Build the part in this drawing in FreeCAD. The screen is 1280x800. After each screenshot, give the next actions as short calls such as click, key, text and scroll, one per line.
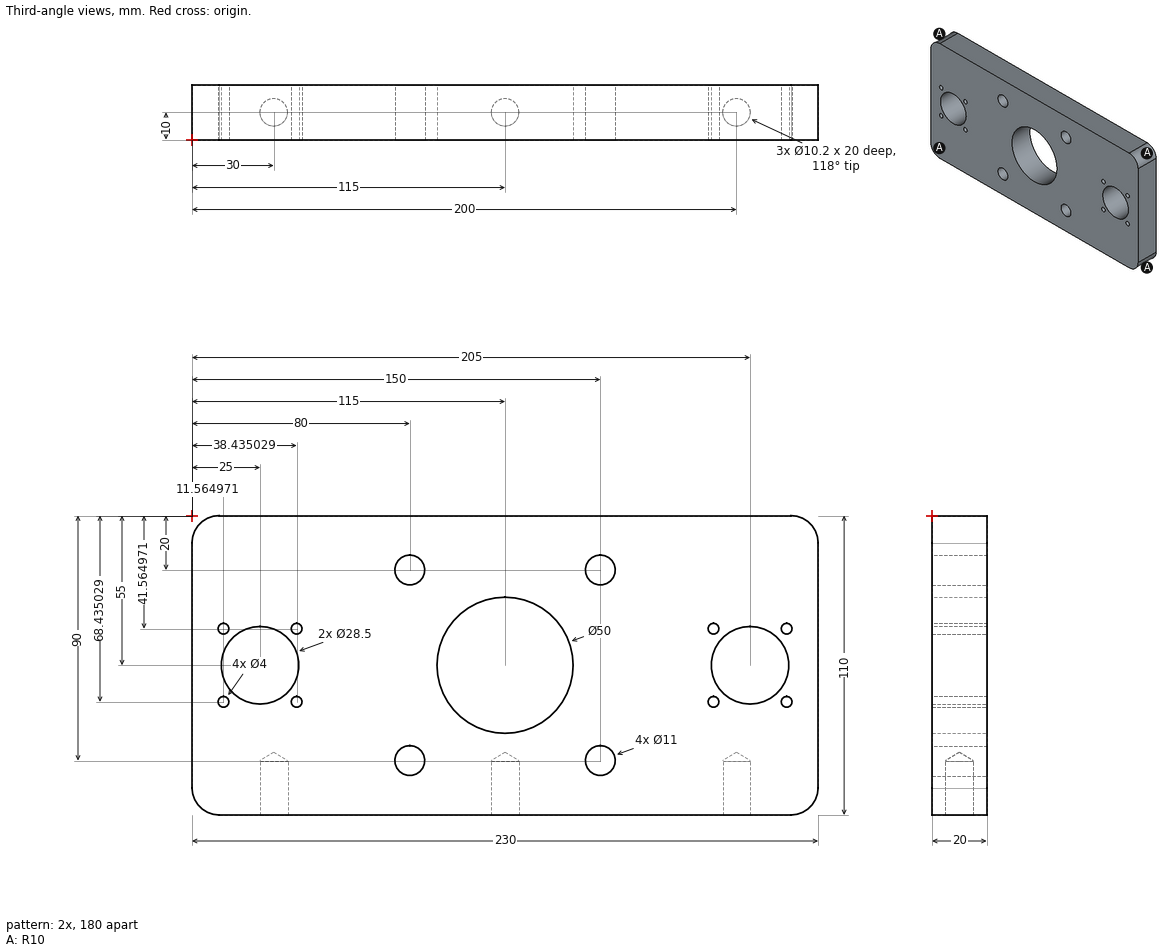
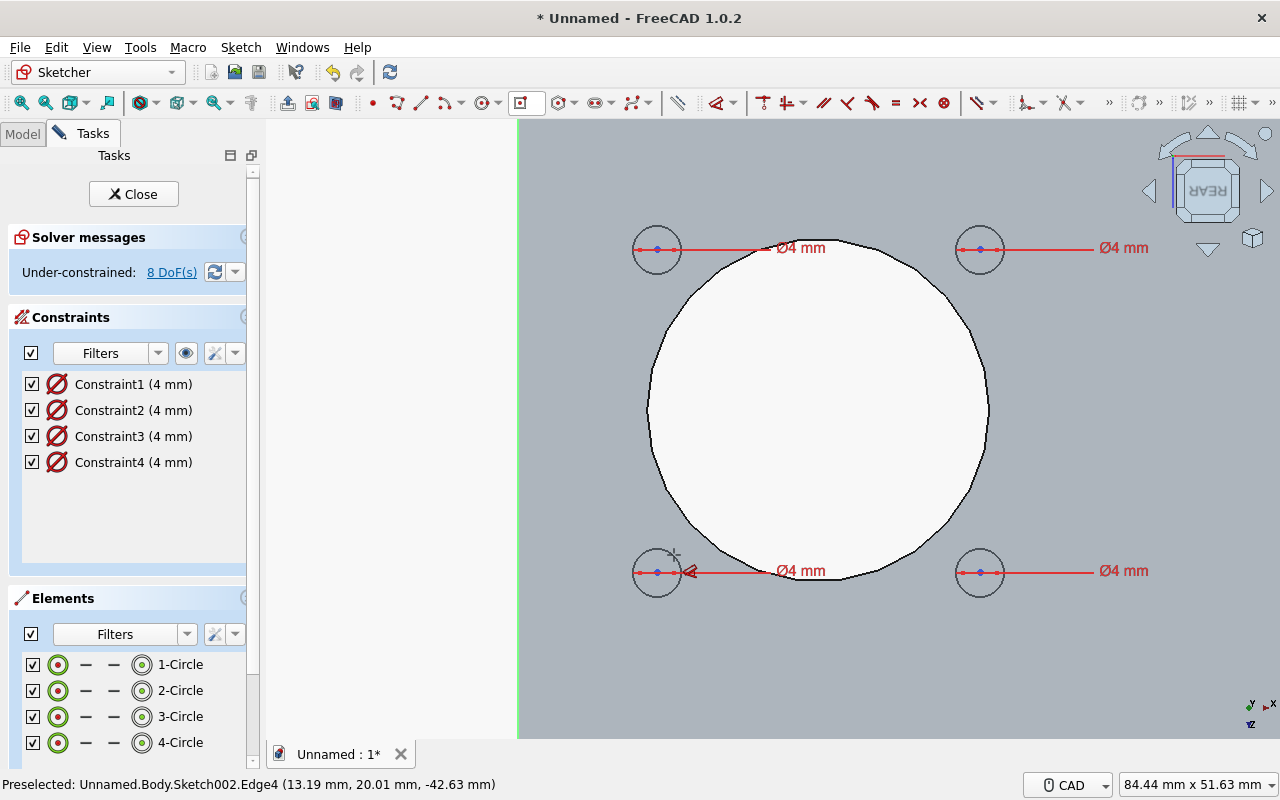
click(657, 250)
click(587, 216)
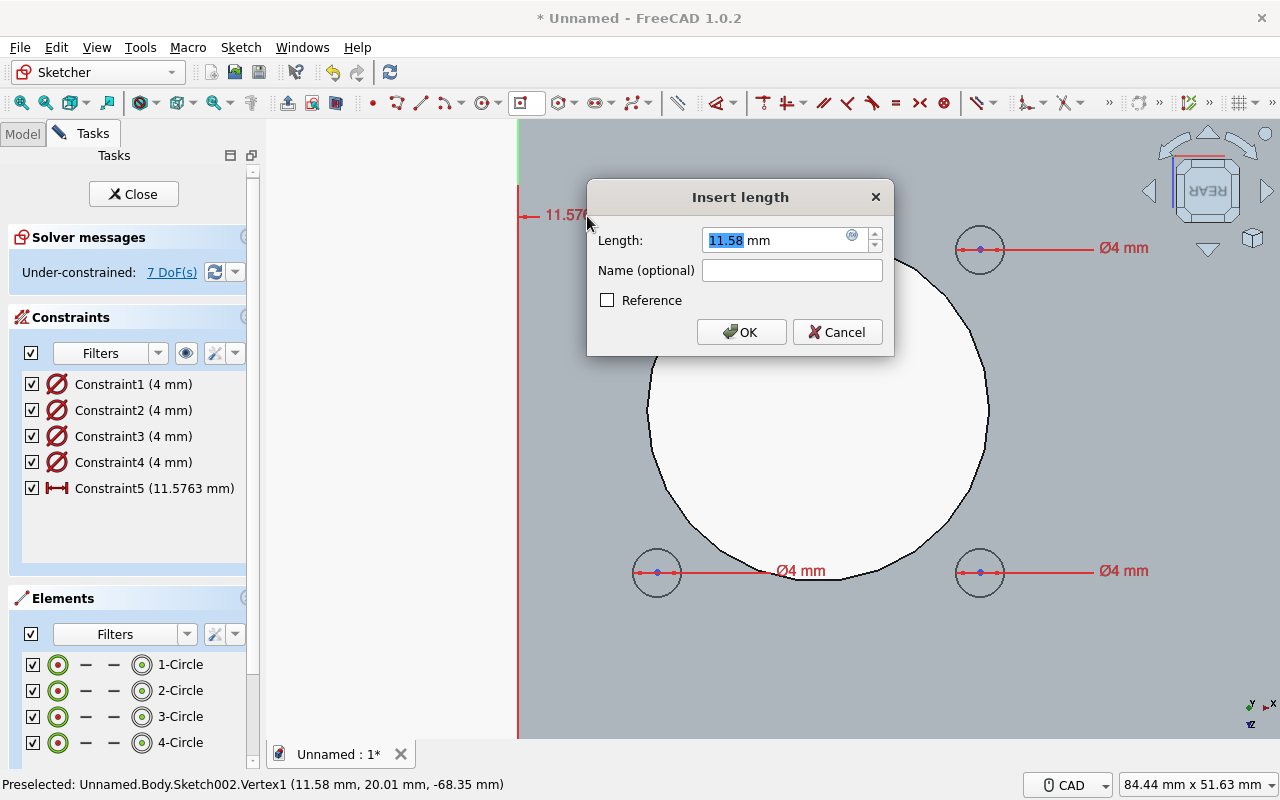
text(11.564971)
key(Return)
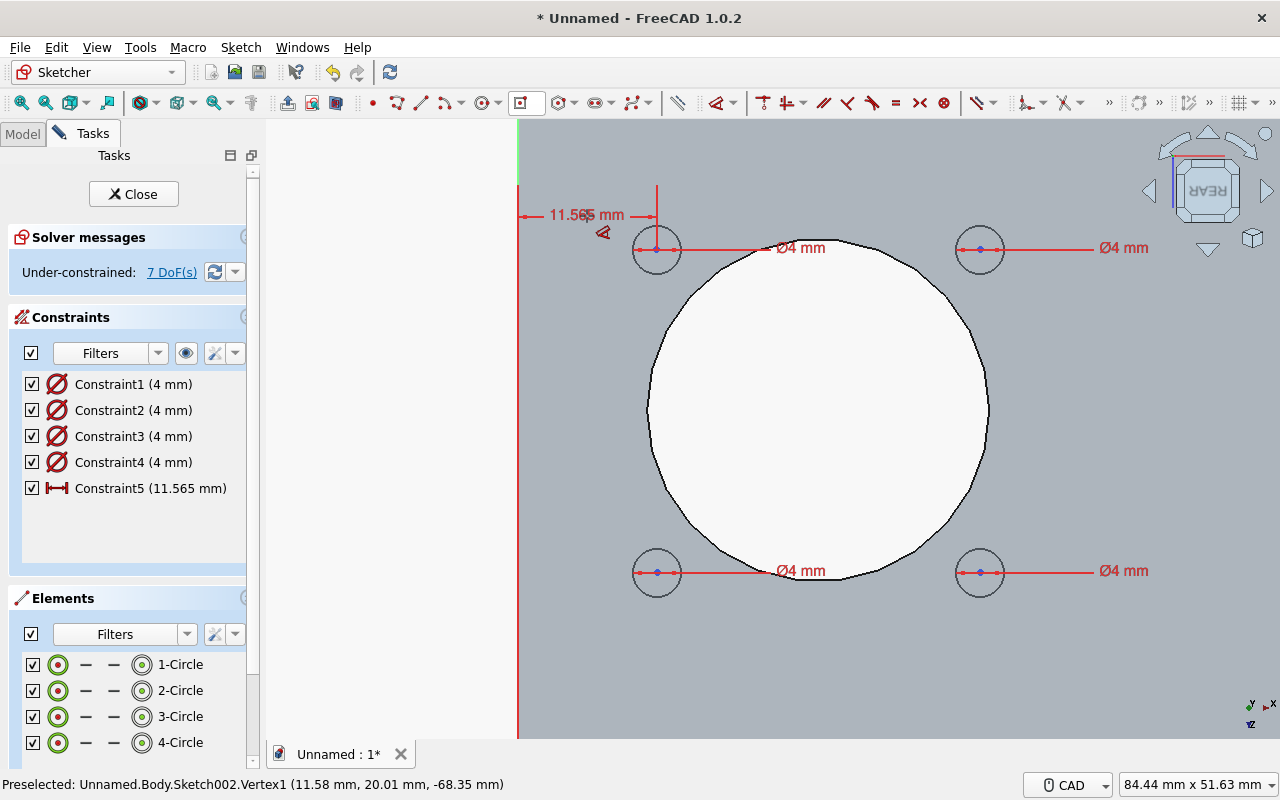
click(657, 250)
click(484, 480)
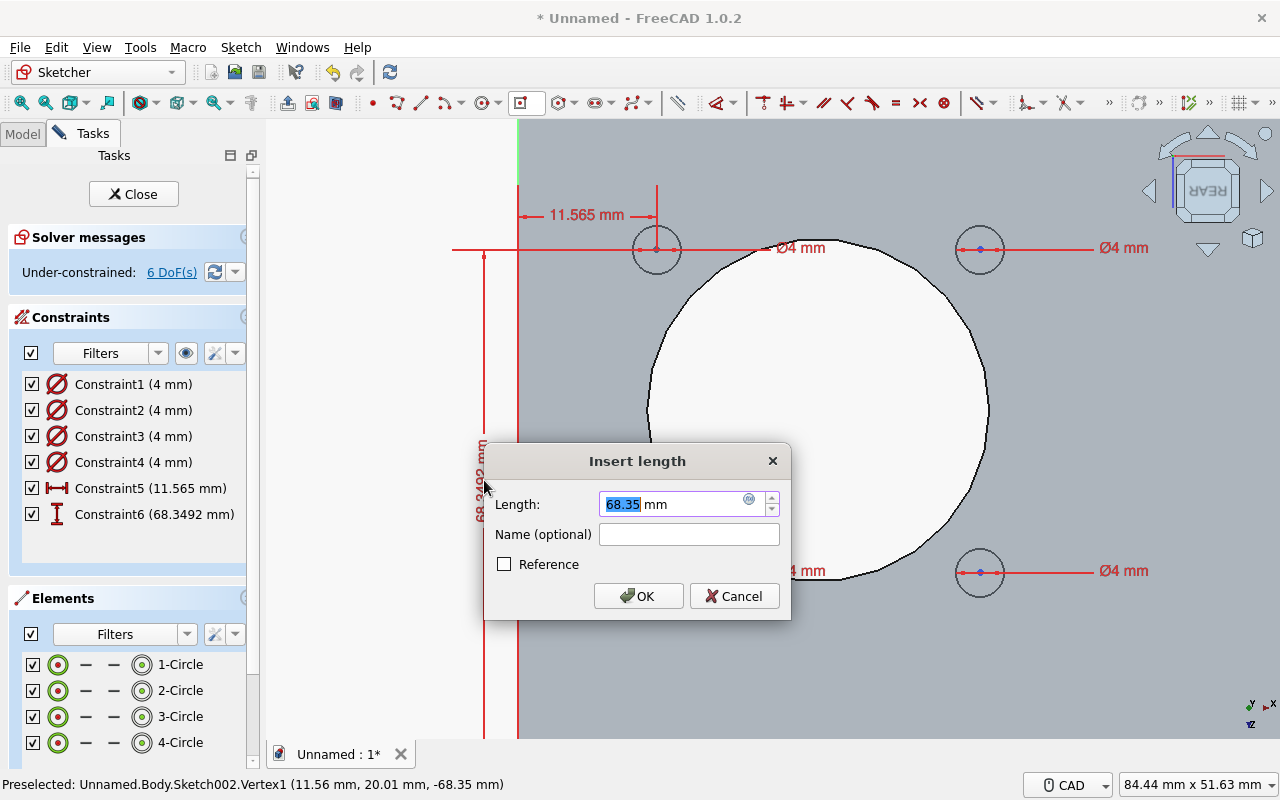
text(68.435029)
key(Return)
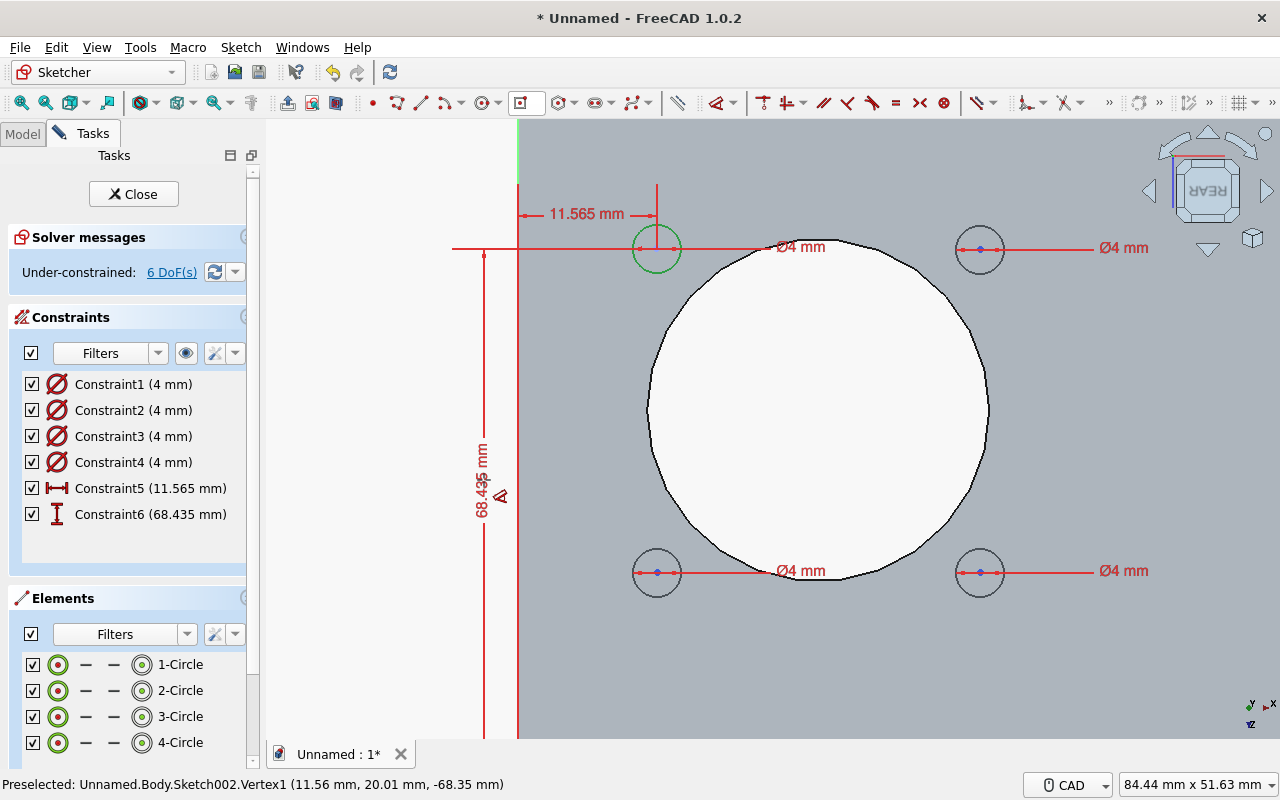
click(980, 250)
click(749, 216)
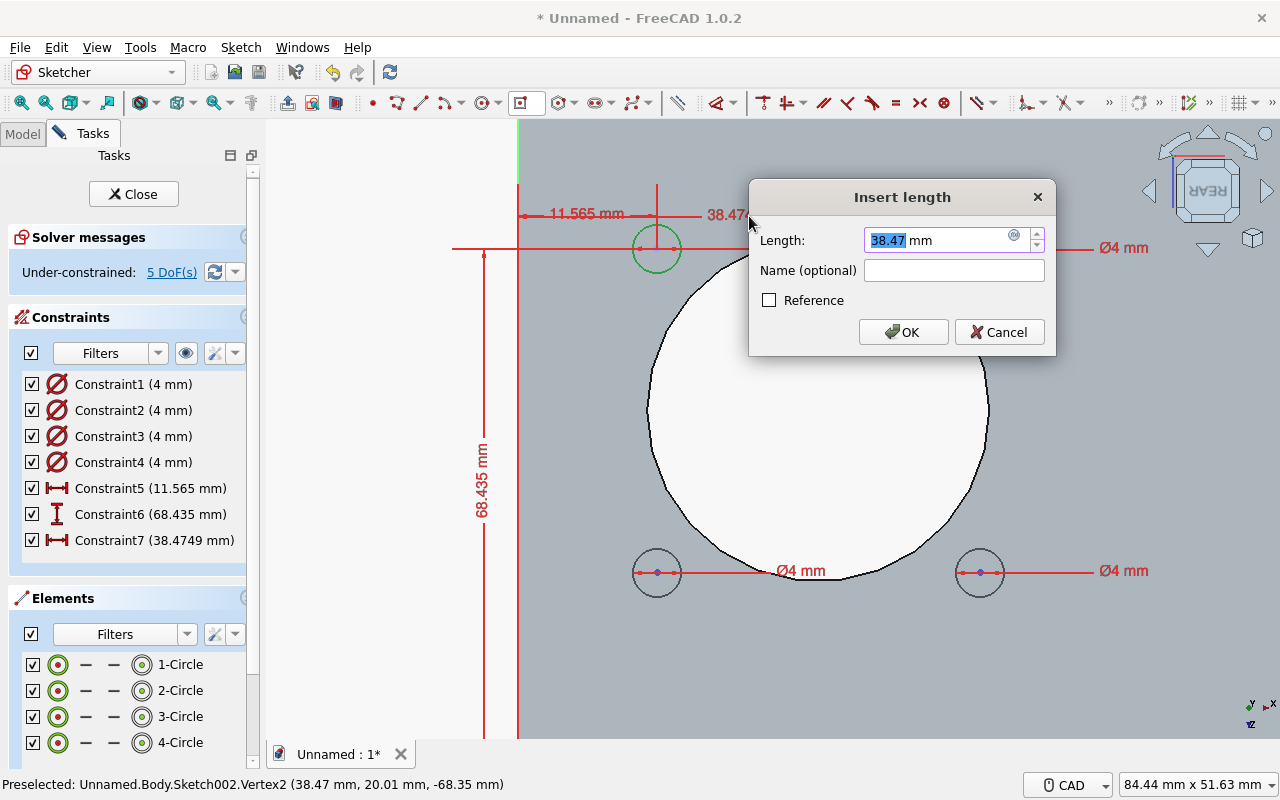
text(38.435029)
key(Return)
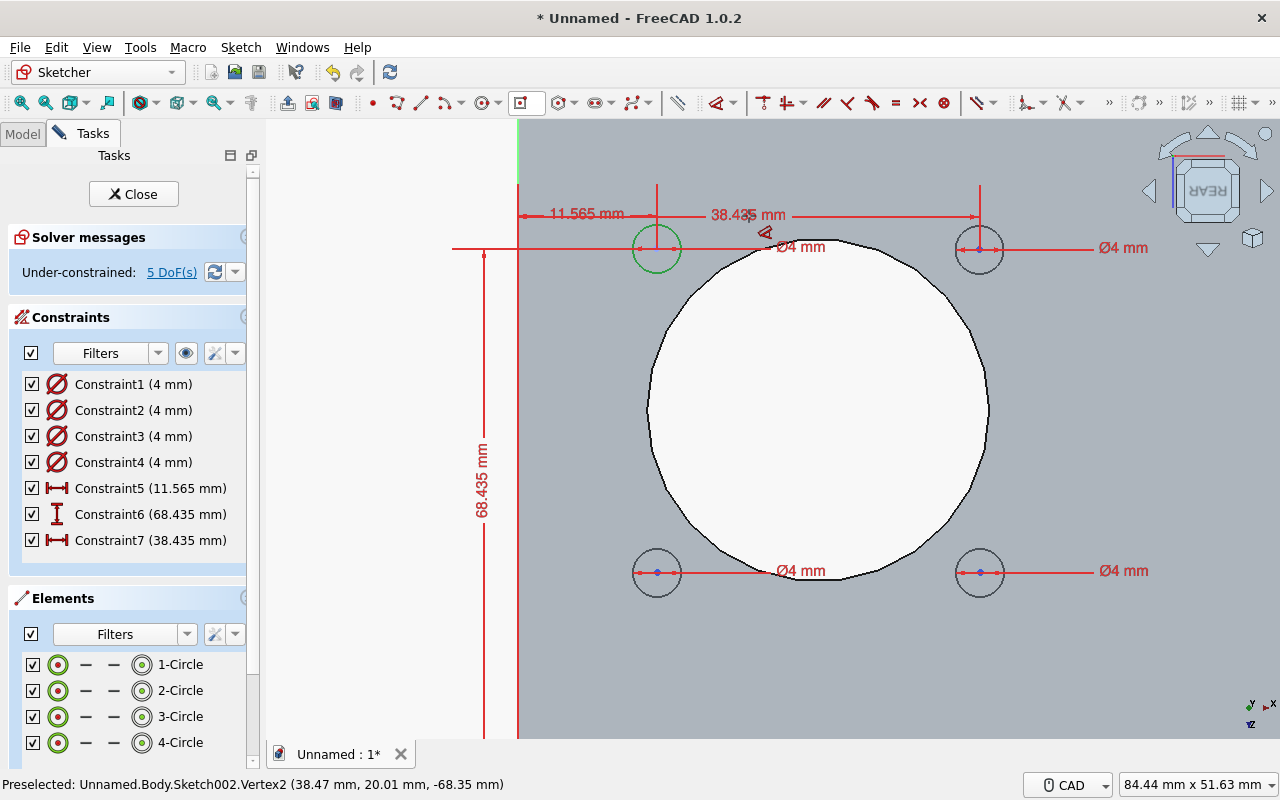
click(980, 250)
click(484, 374)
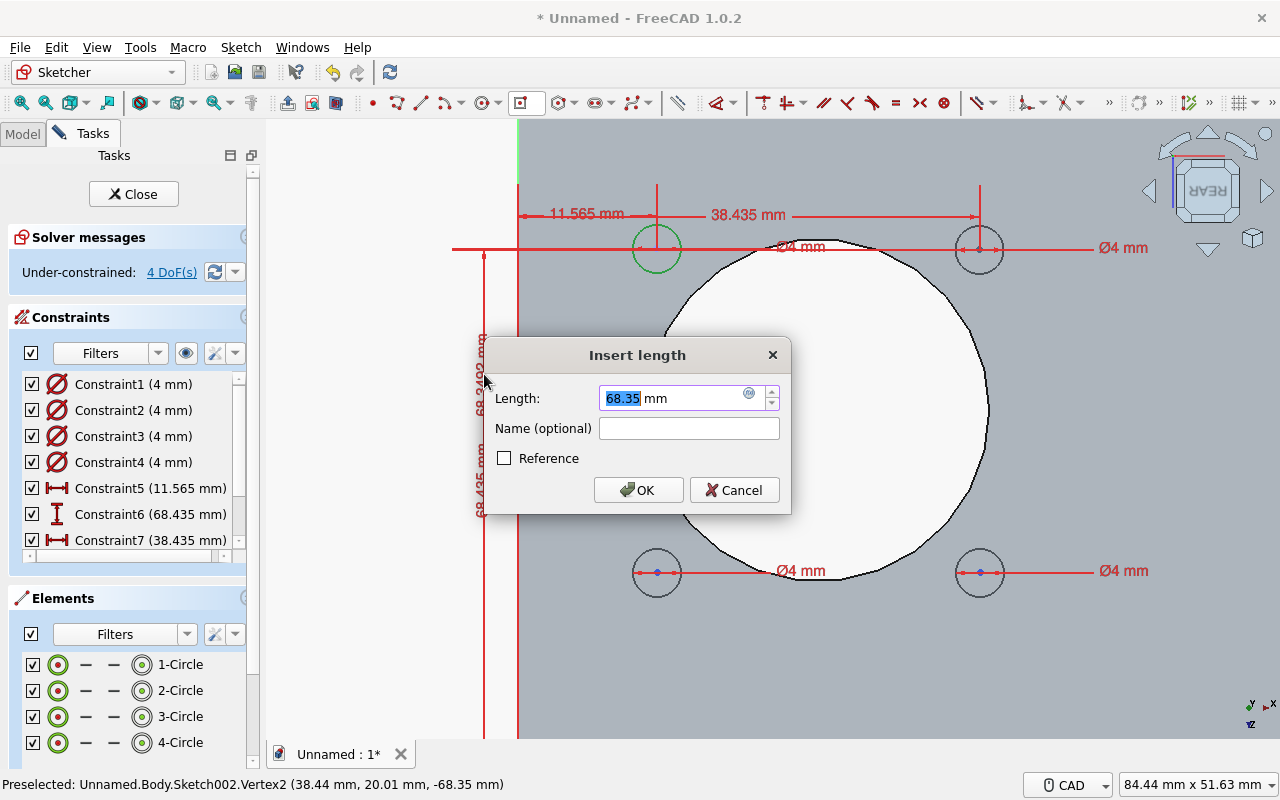
text(68.435029)
key(Return)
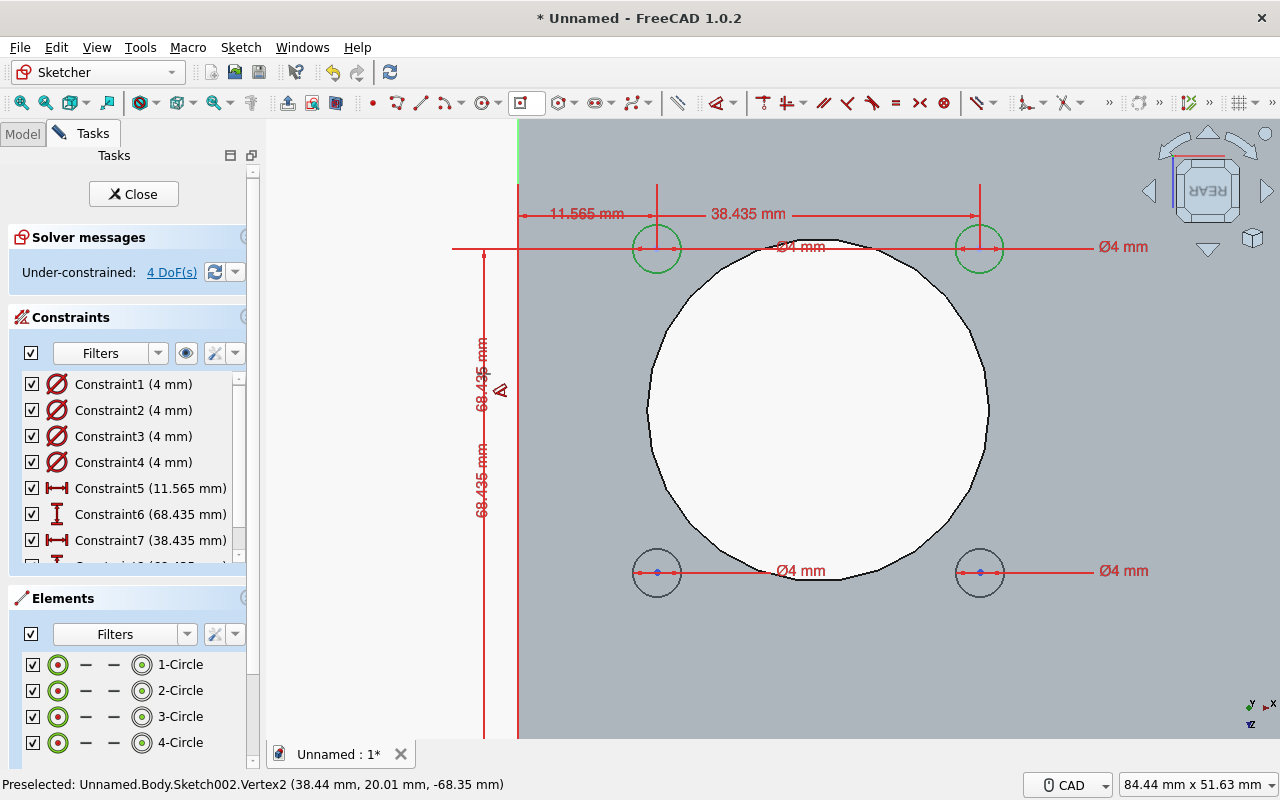
click(980, 573)
click(749, 539)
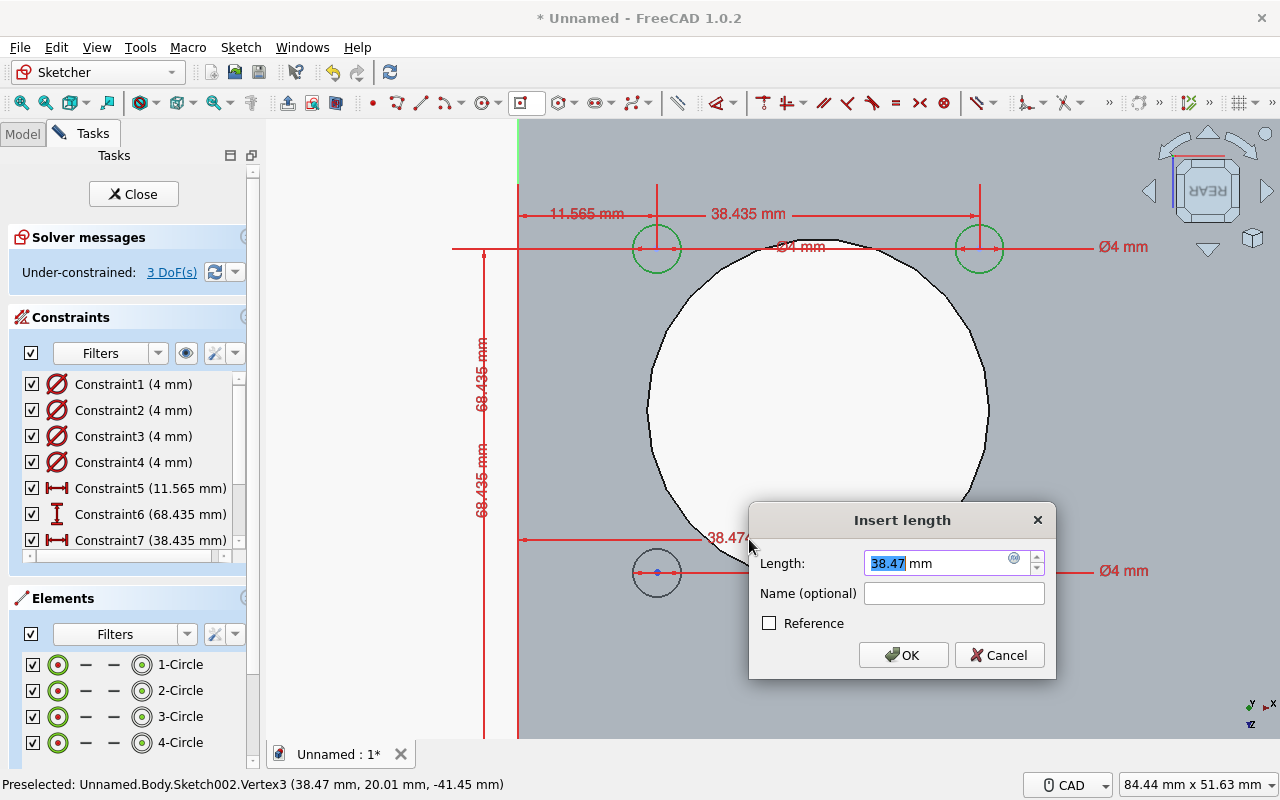
text(38.435029)
key(Return)